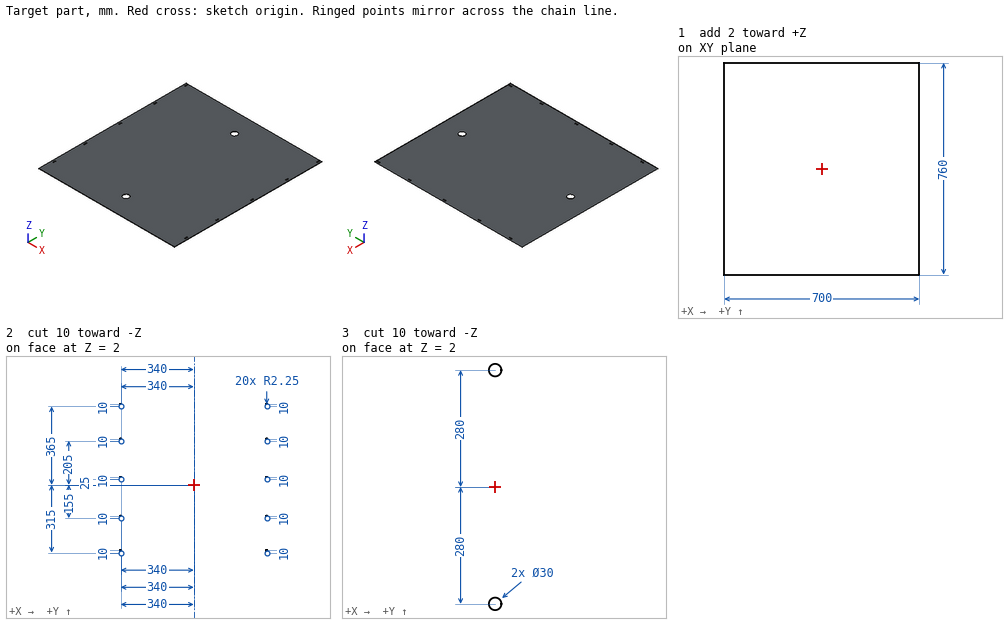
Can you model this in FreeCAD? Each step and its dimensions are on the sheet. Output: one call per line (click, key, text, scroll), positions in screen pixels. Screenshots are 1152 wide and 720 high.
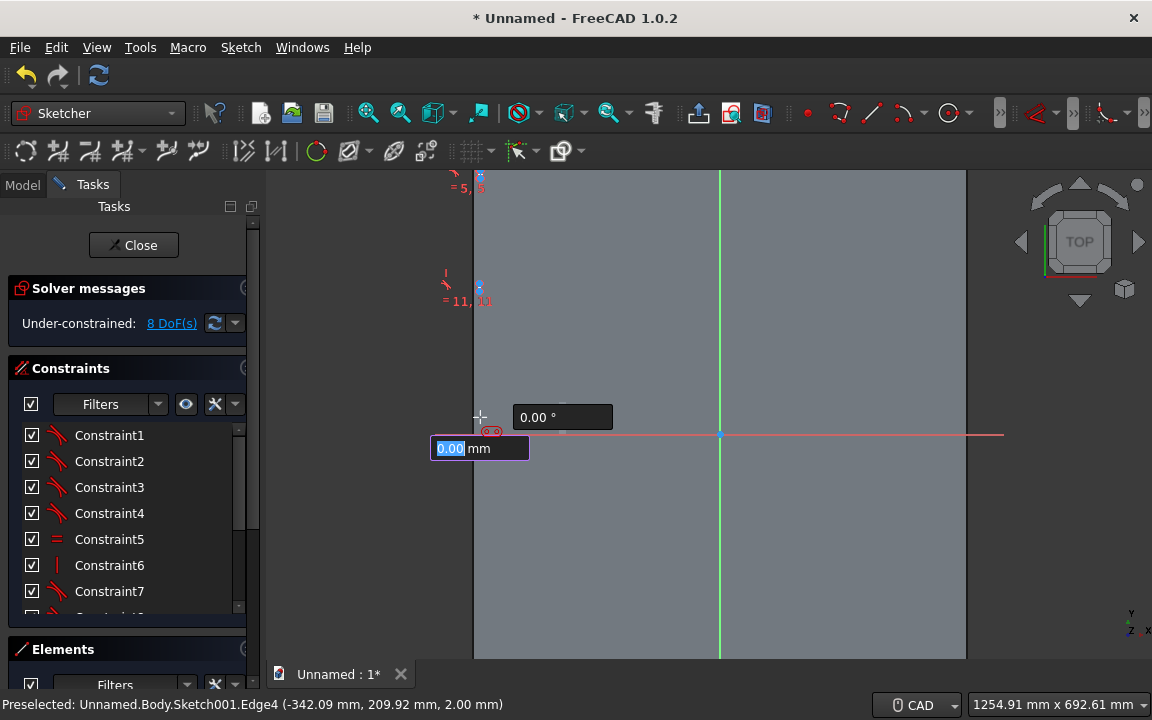
scroll(480, 410, up, 5)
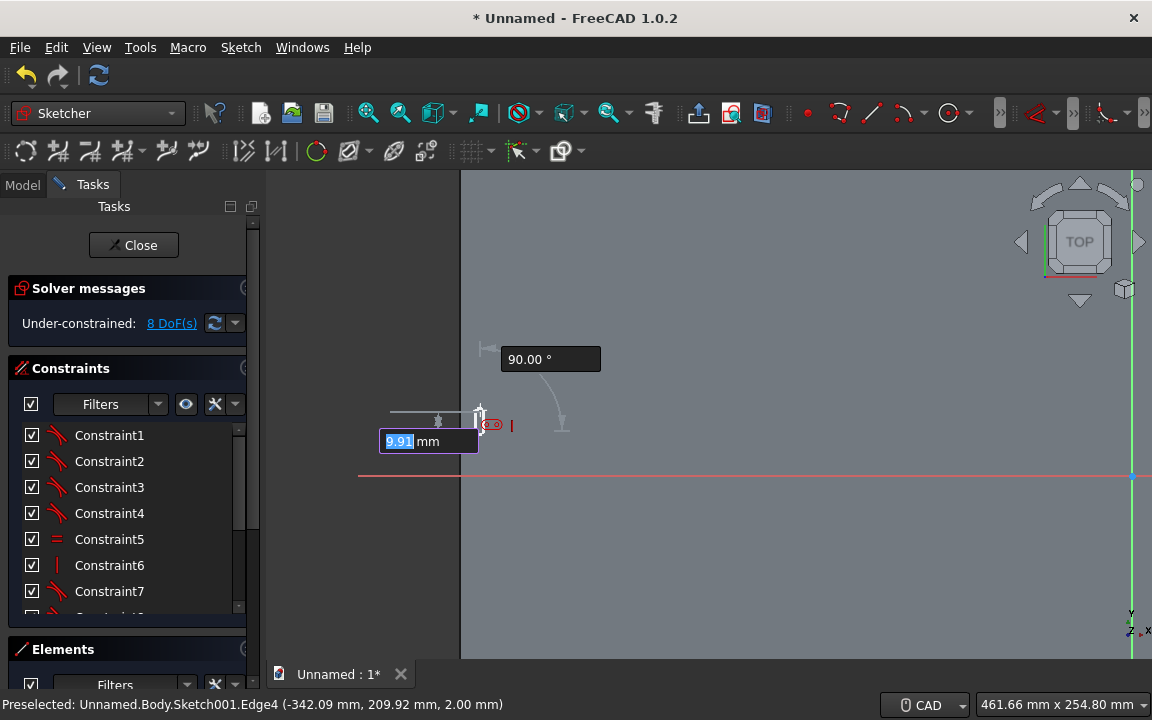
click(480, 409)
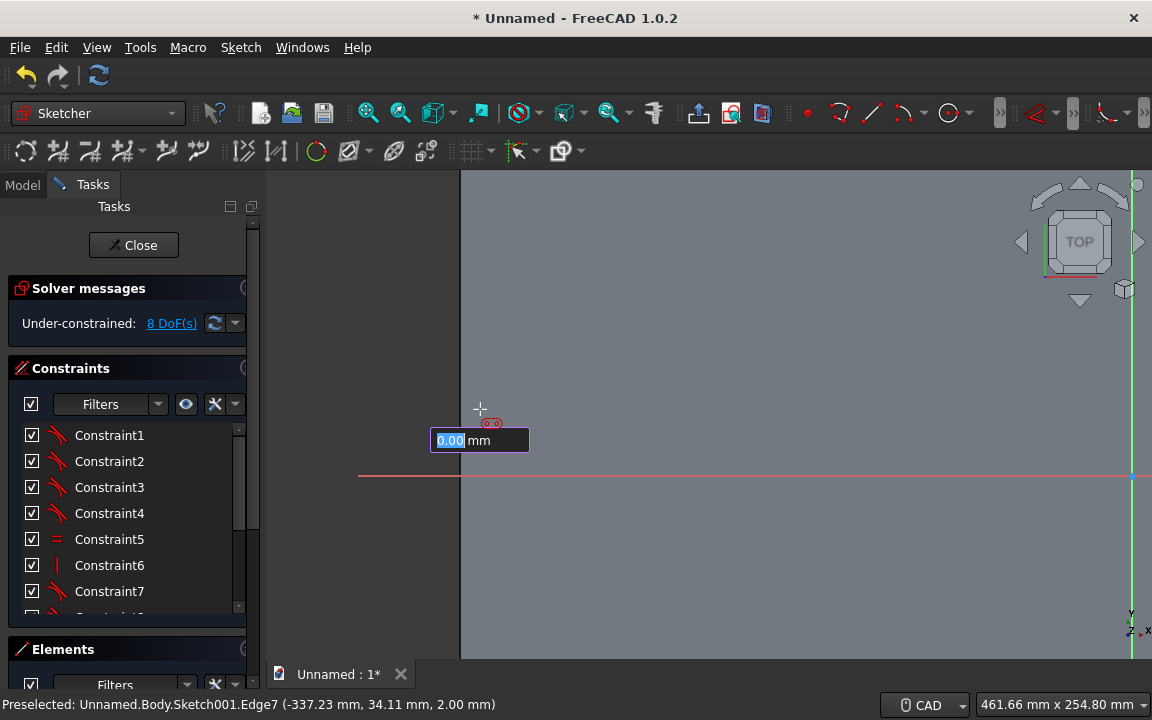
scroll(475, 418, up, 7)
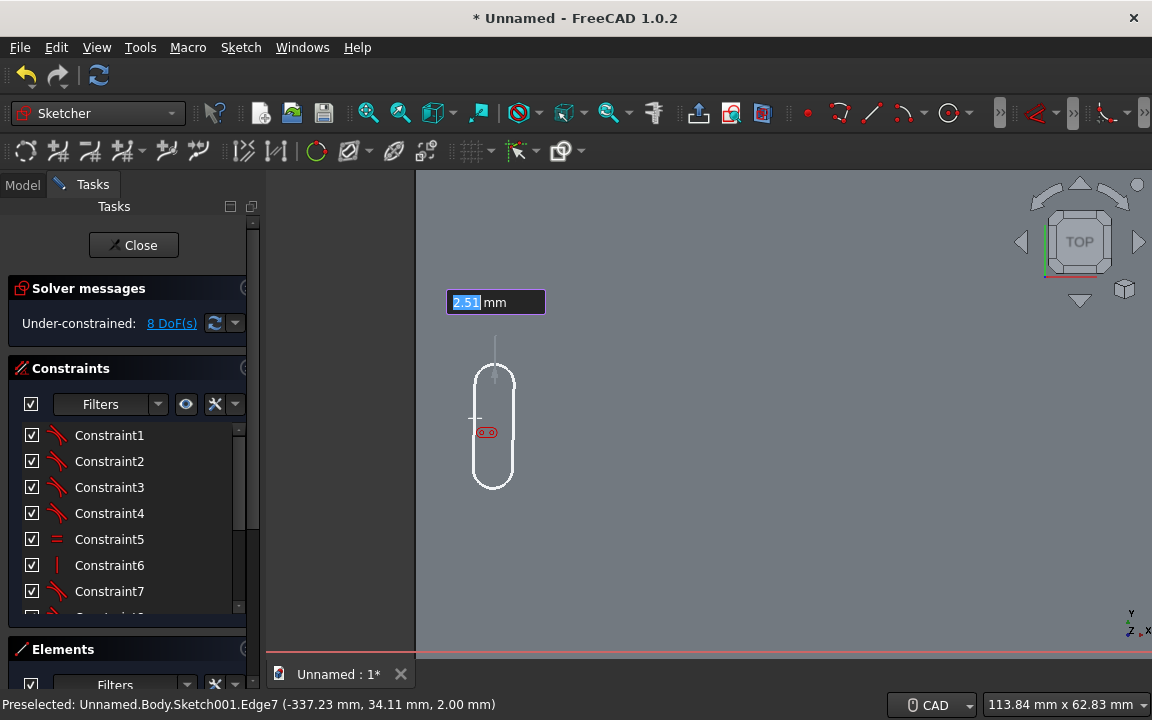
click(476, 418)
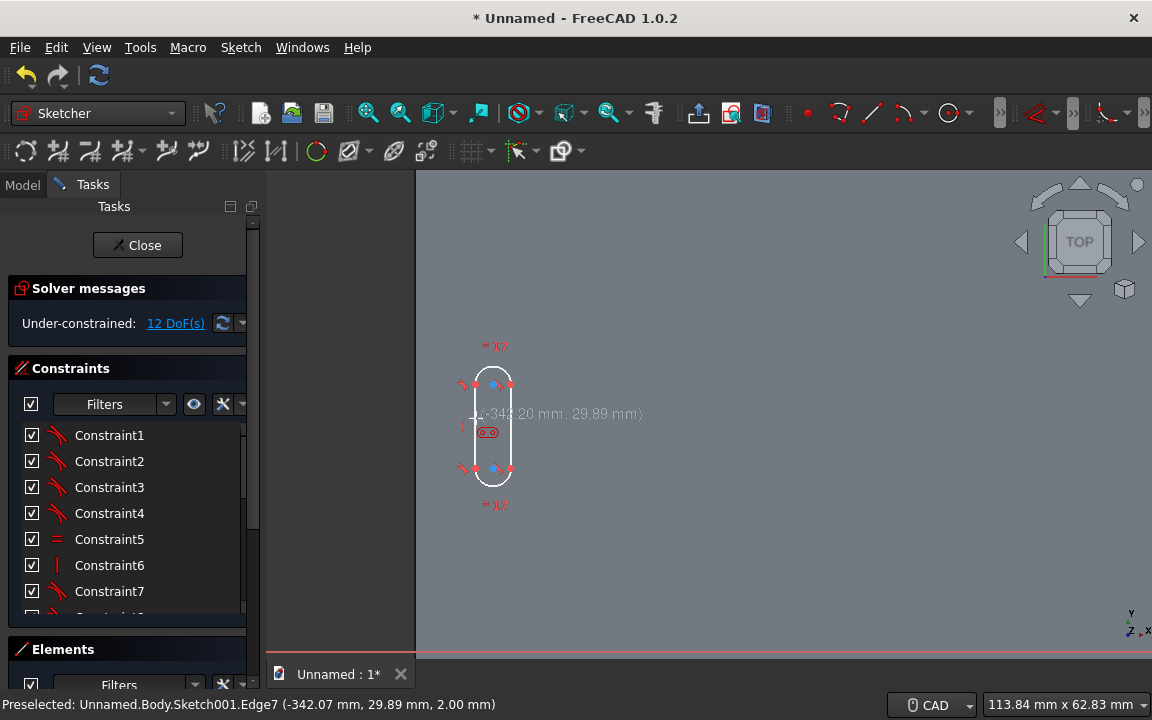
scroll(479, 414, down, 14)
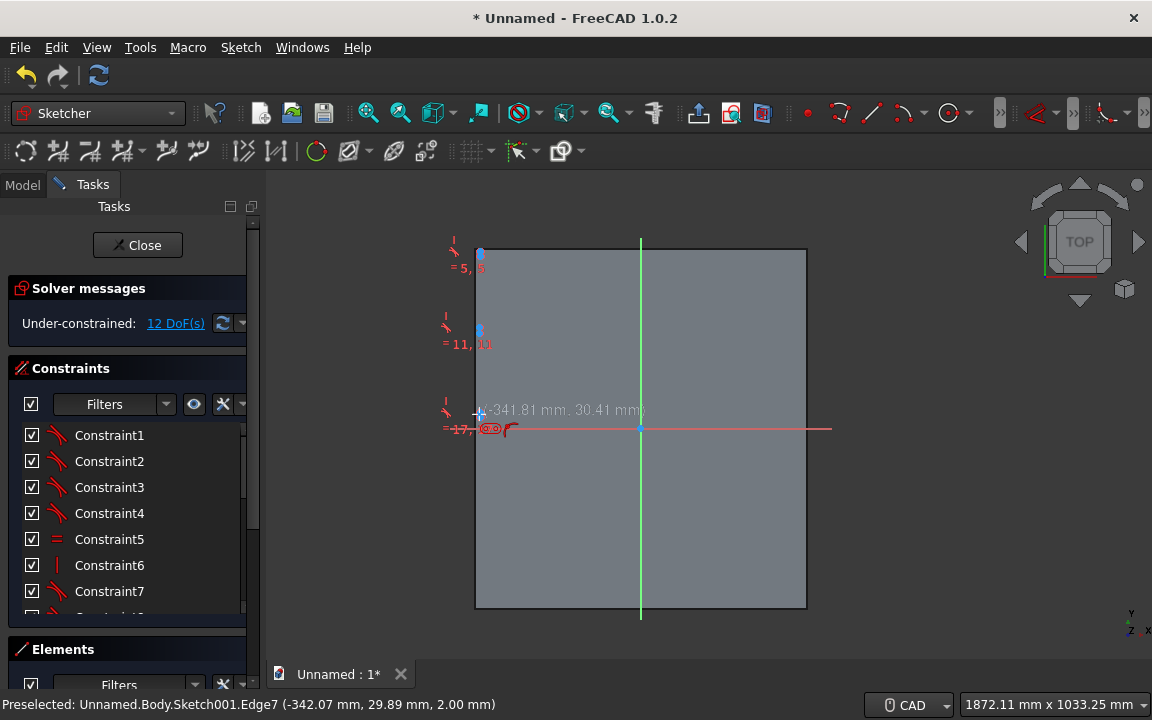
scroll(802, 256, up, 16)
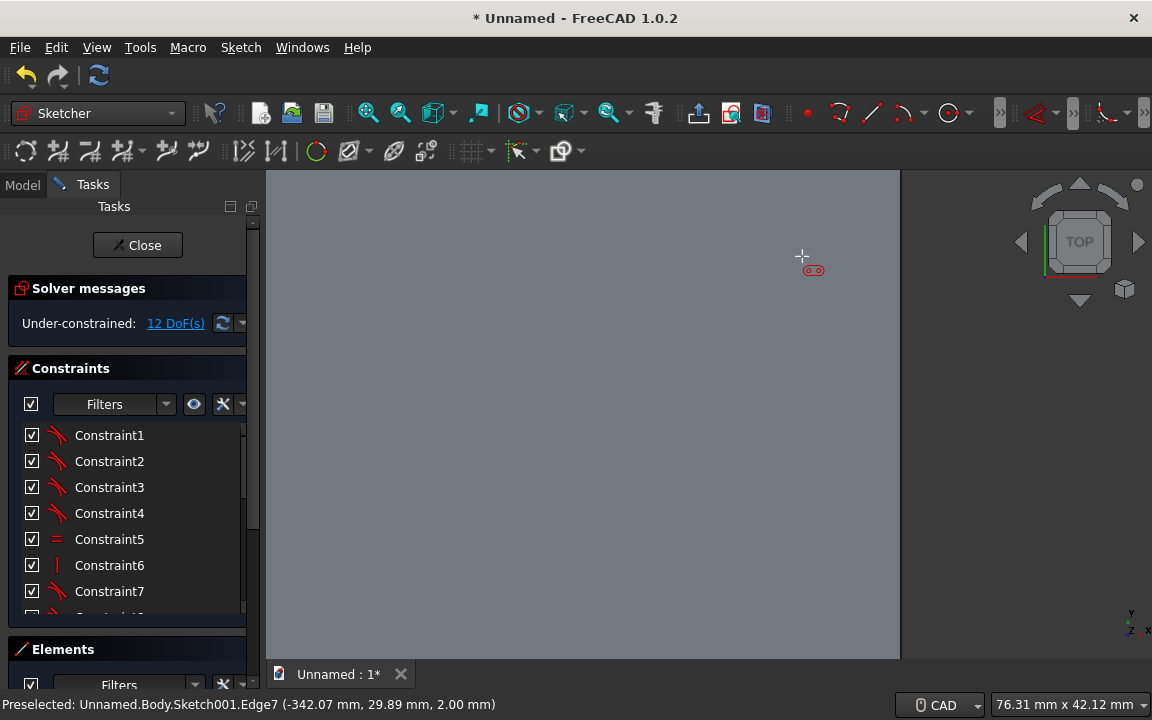
scroll(802, 256, down, 16)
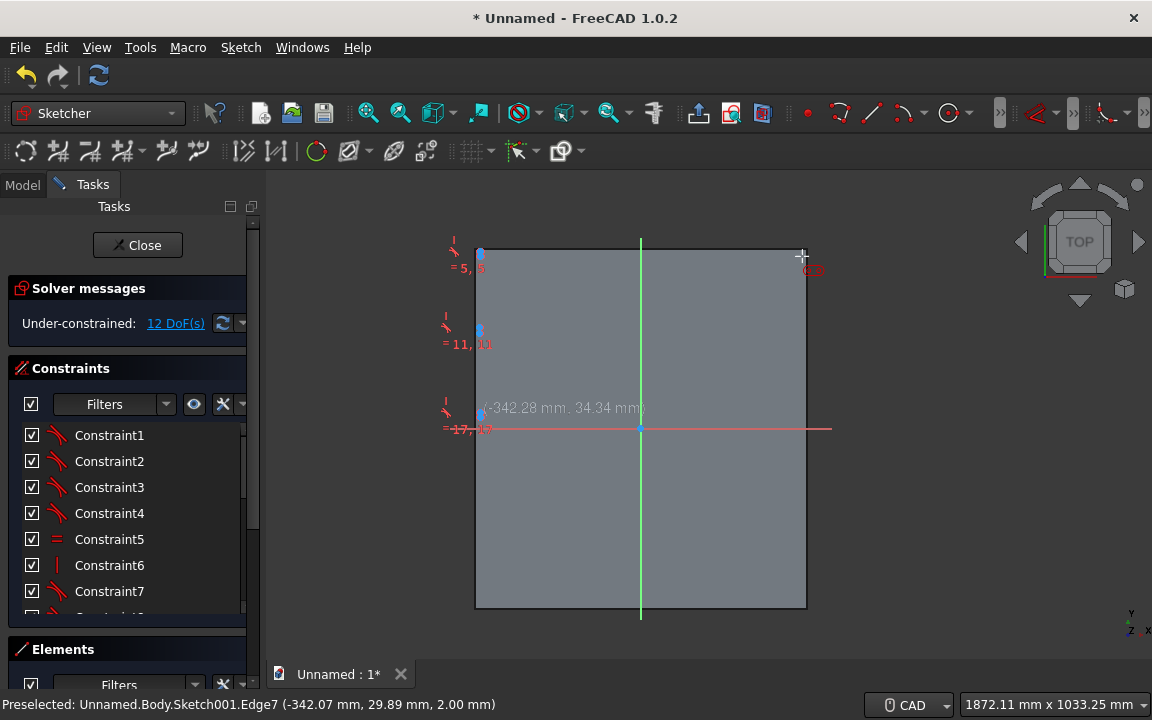
click(802, 256)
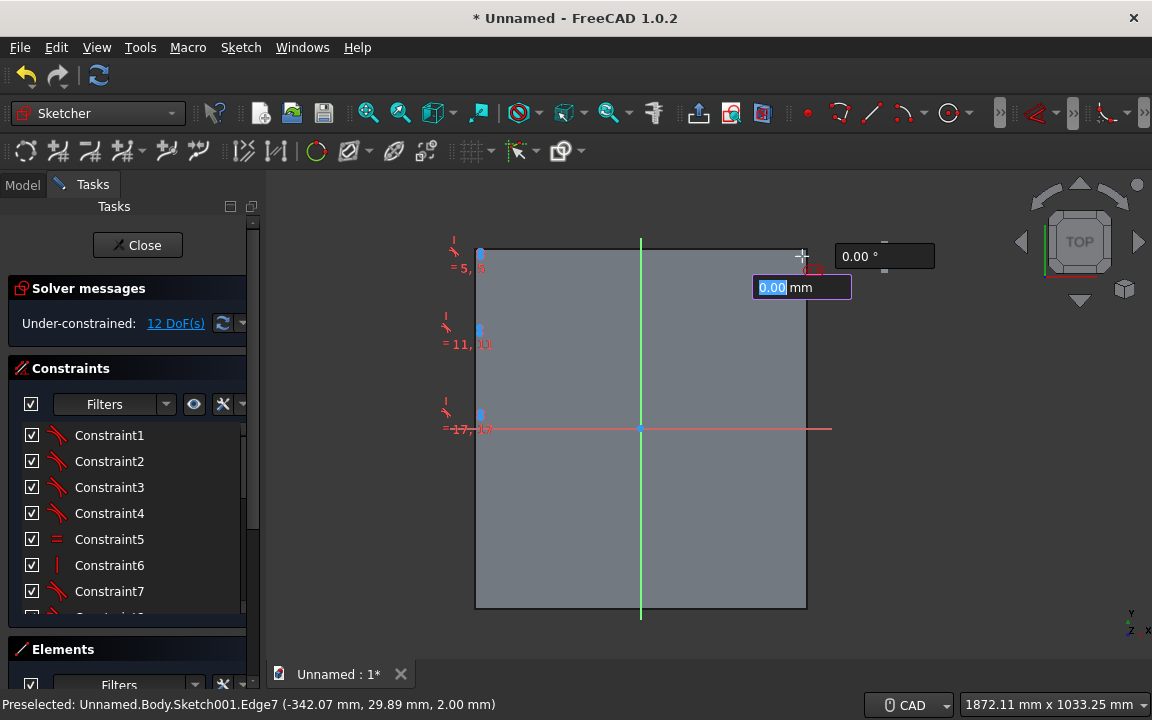
scroll(802, 251, up, 7)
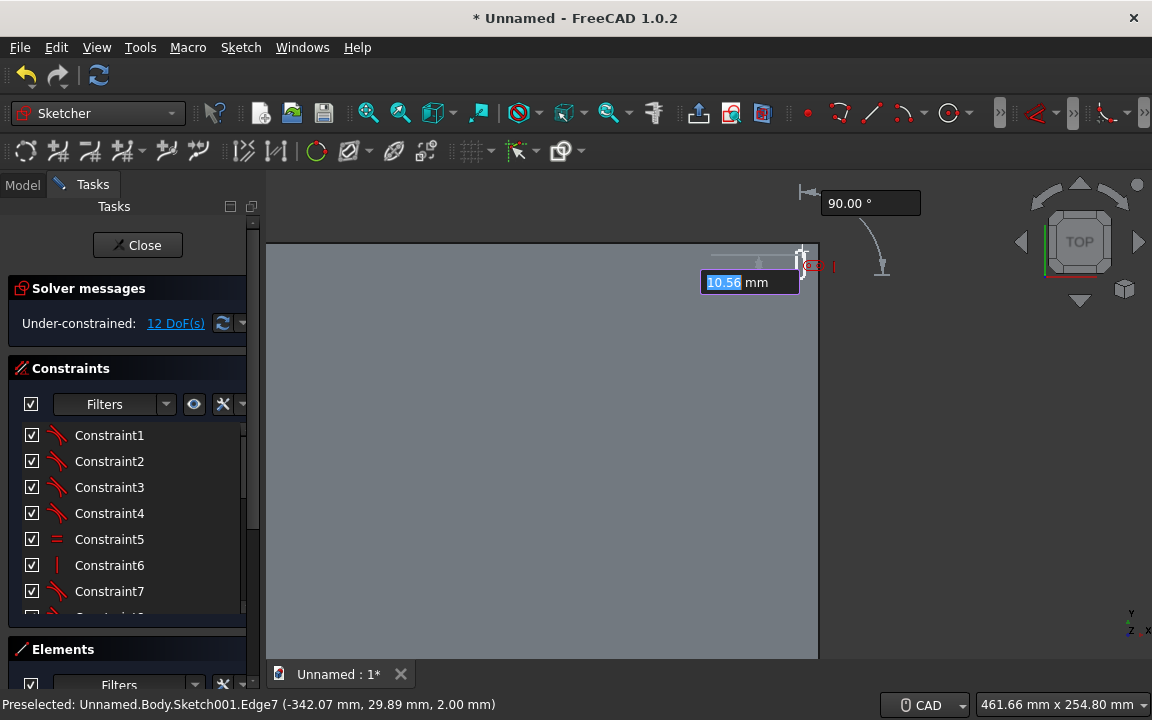
click(800, 252)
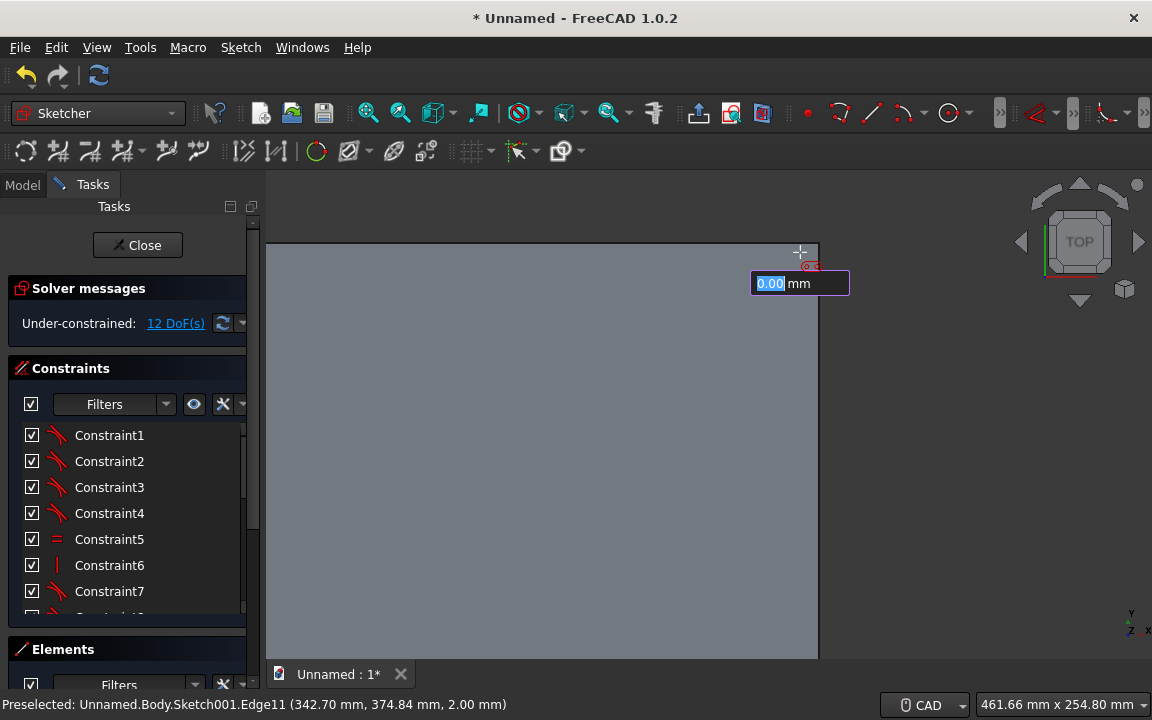
scroll(795, 262, up, 7)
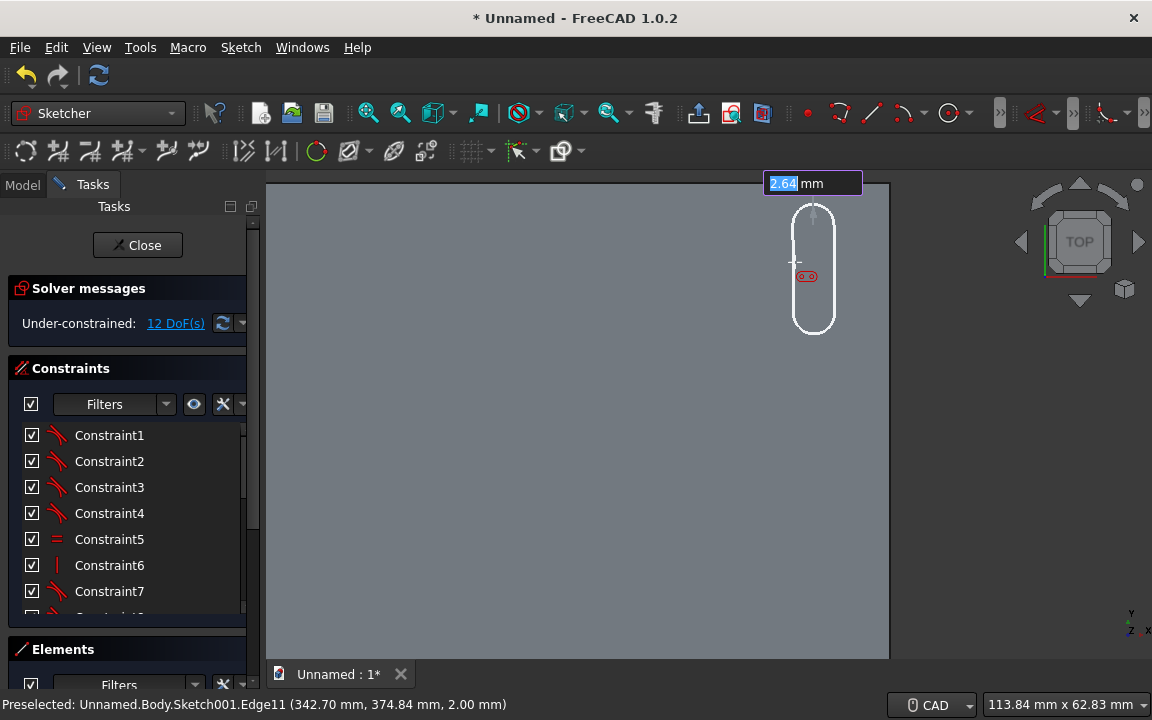
click(795, 261)